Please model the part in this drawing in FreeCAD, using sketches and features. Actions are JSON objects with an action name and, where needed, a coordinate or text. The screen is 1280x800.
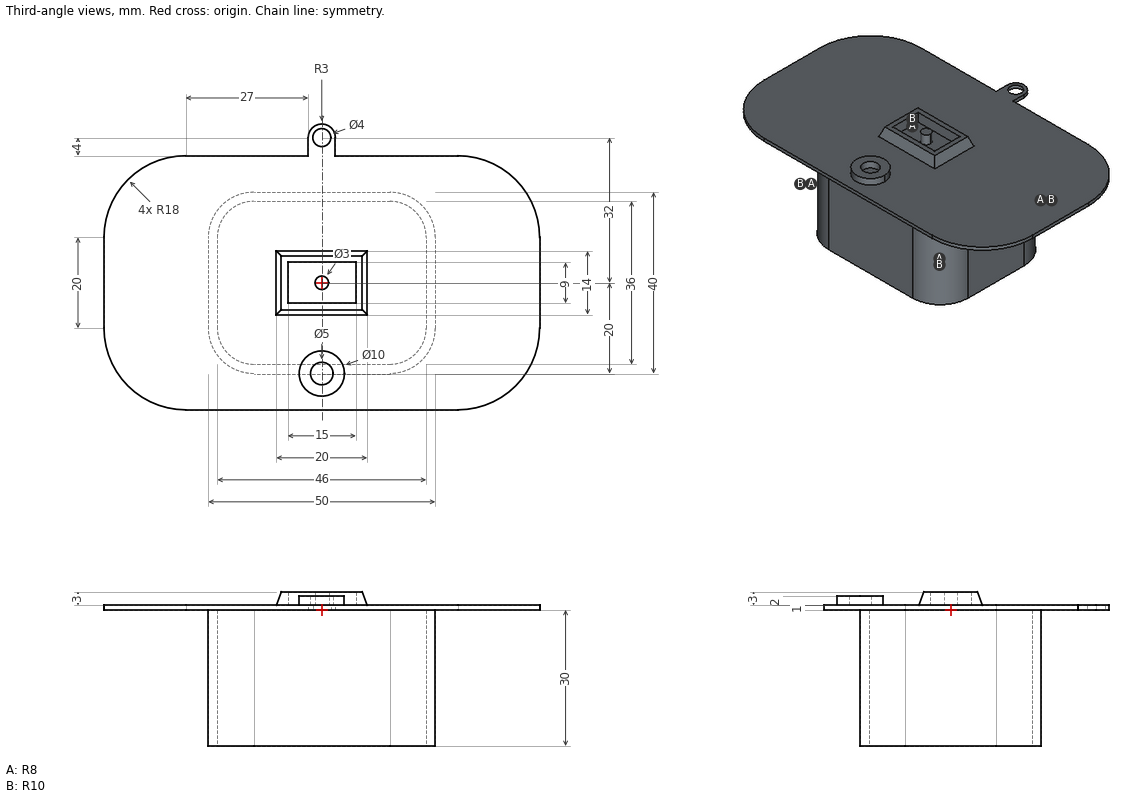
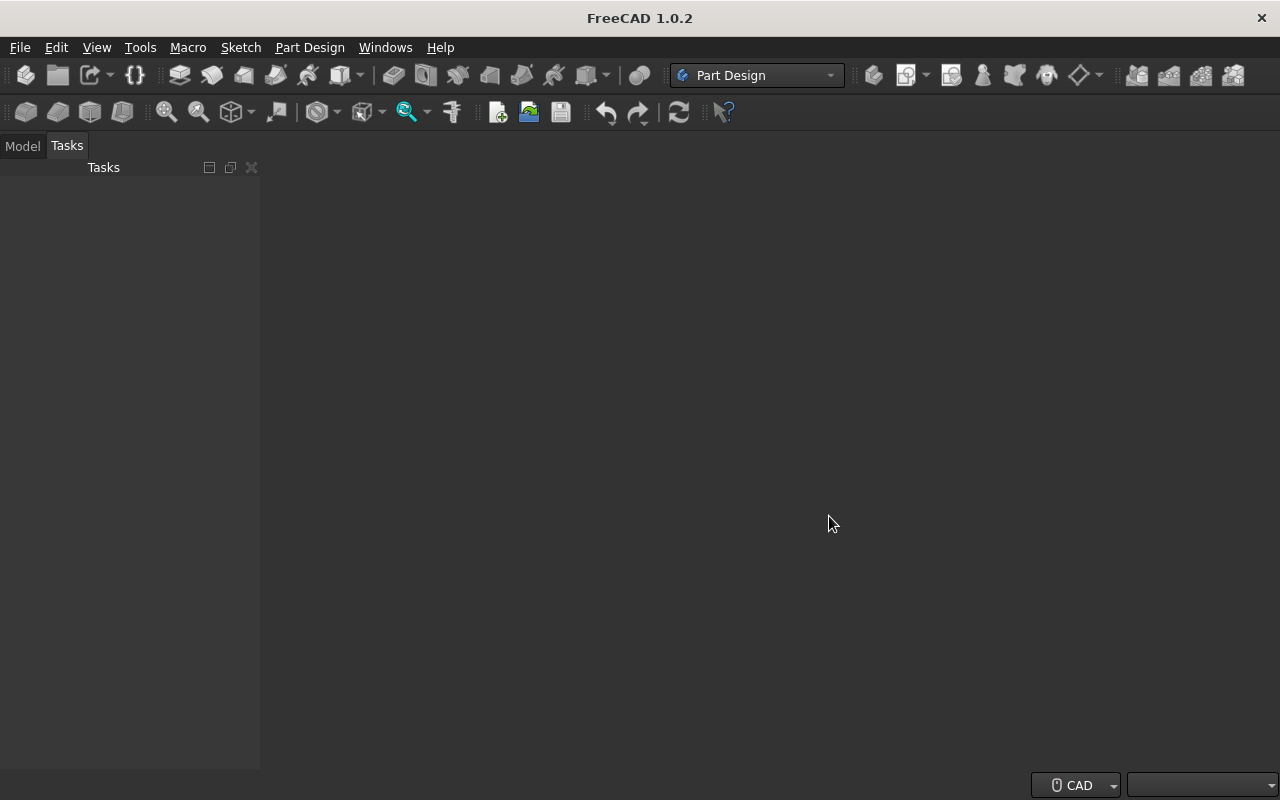
{"action": "left_click", "coordinate": [498, 112]}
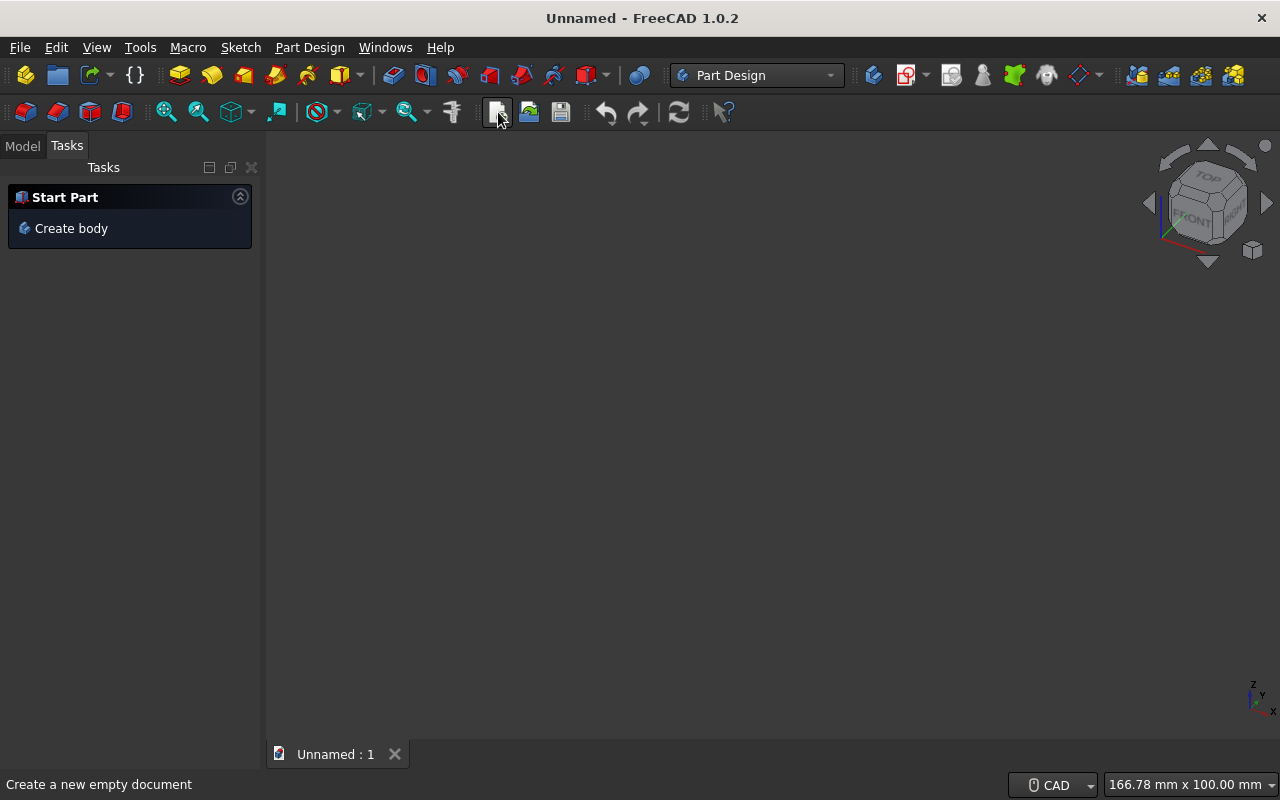
{"action": "left_click", "coordinate": [906, 76]}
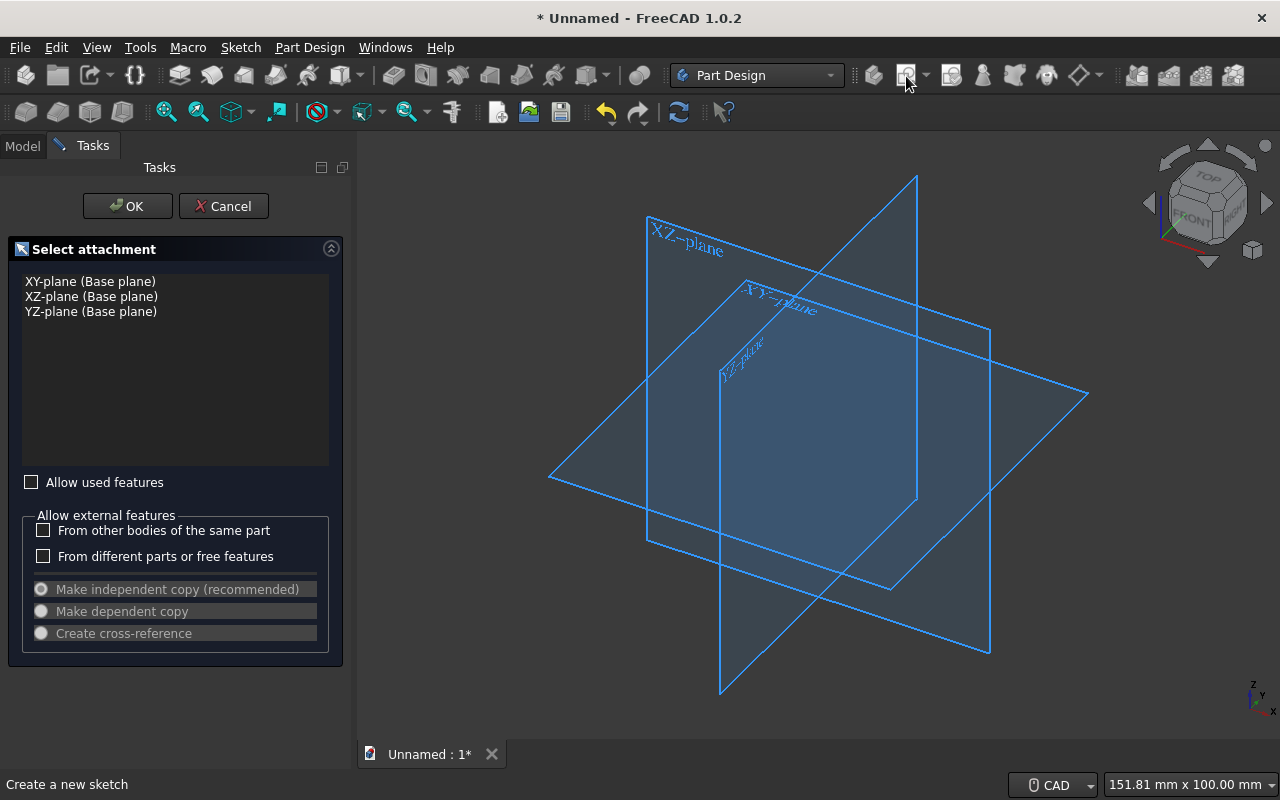
{"action": "left_click", "coordinate": [82, 282]}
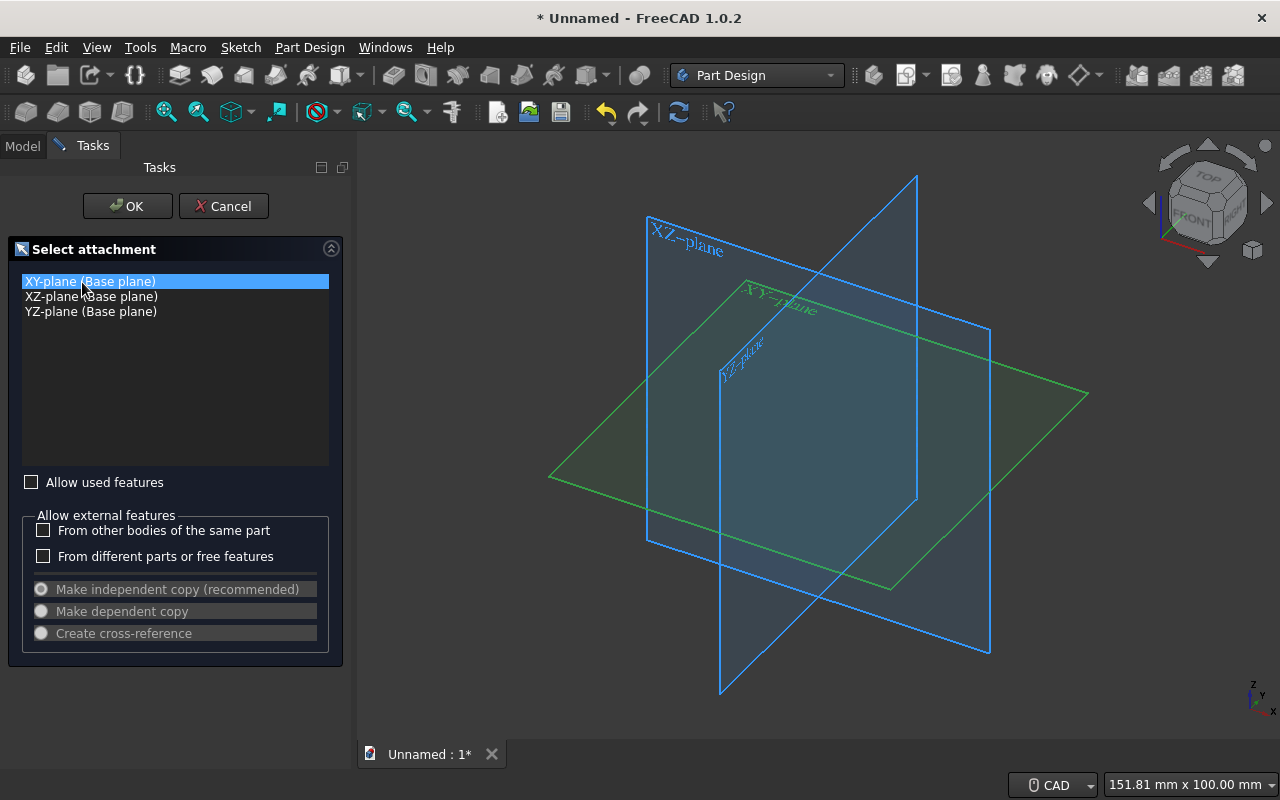
{"action": "left_click", "coordinate": [128, 206]}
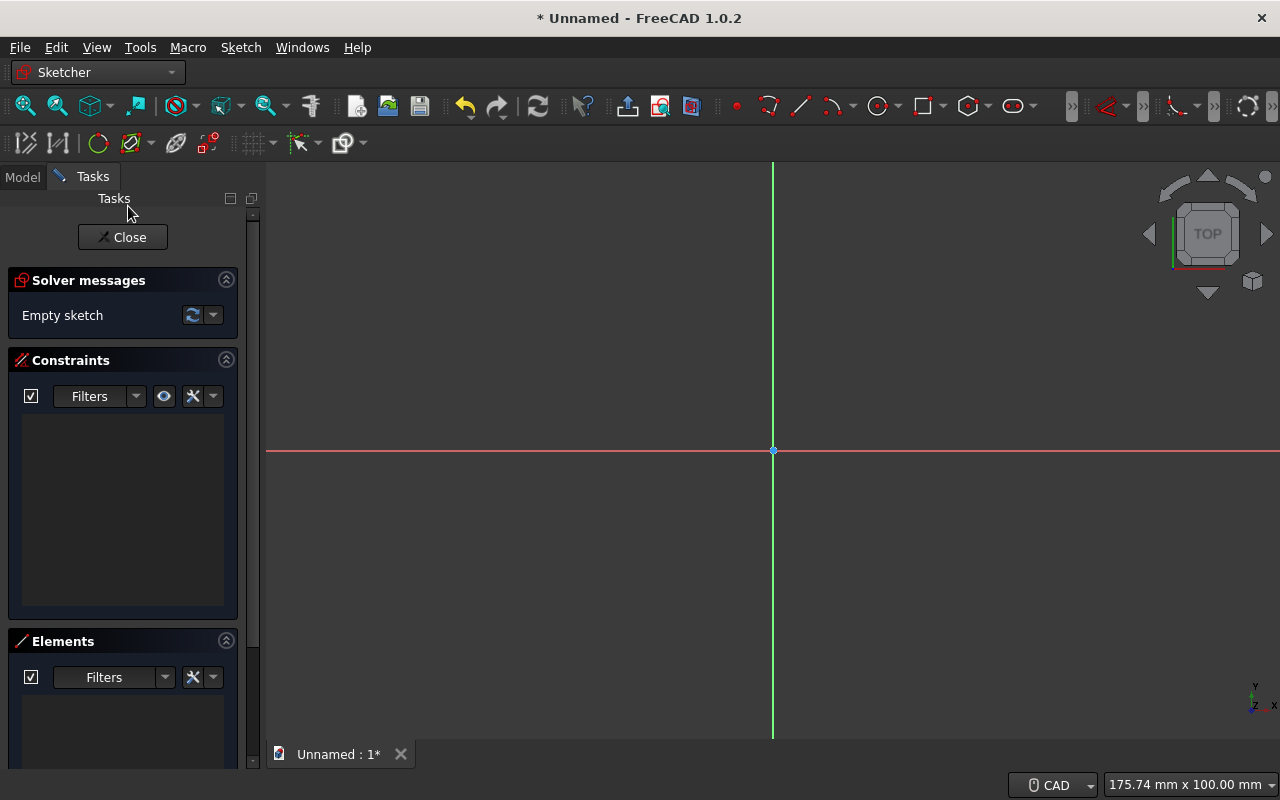
{"action": "left_click", "coordinate": [770, 106]}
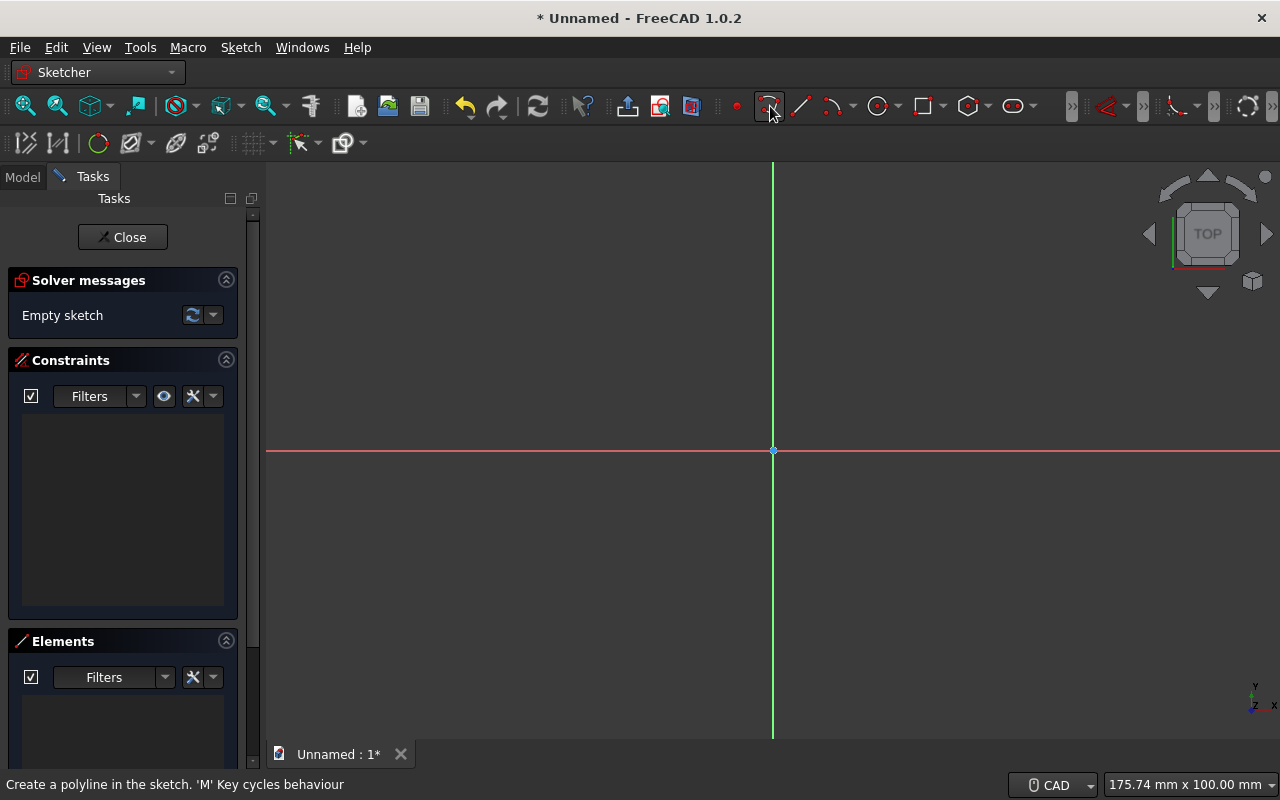
{"action": "left_click", "coordinate": [756, 266]}
{"action": "left_click", "coordinate": [756, 289]}
{"action": "left_click", "coordinate": [600, 289]}
{"action": "right_click", "coordinate": [600, 289]}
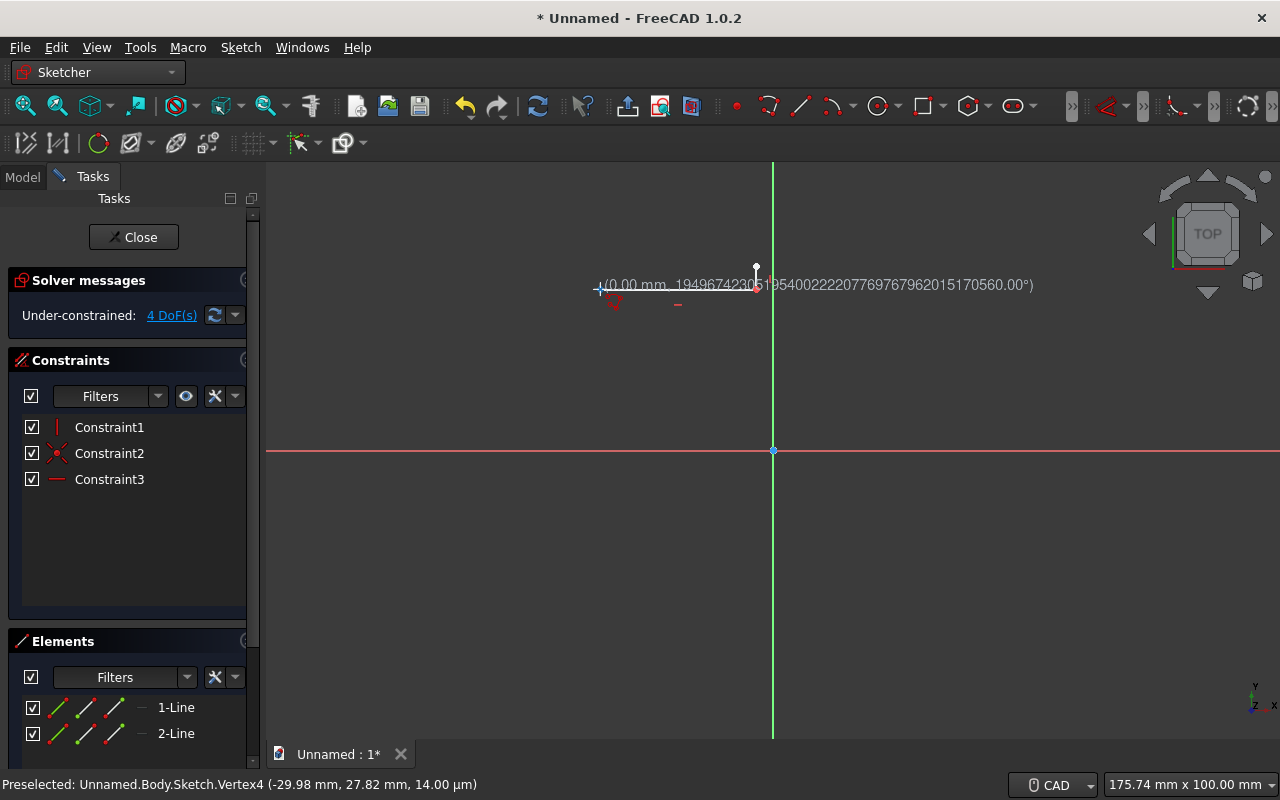
{"action": "left_click", "coordinate": [802, 106]}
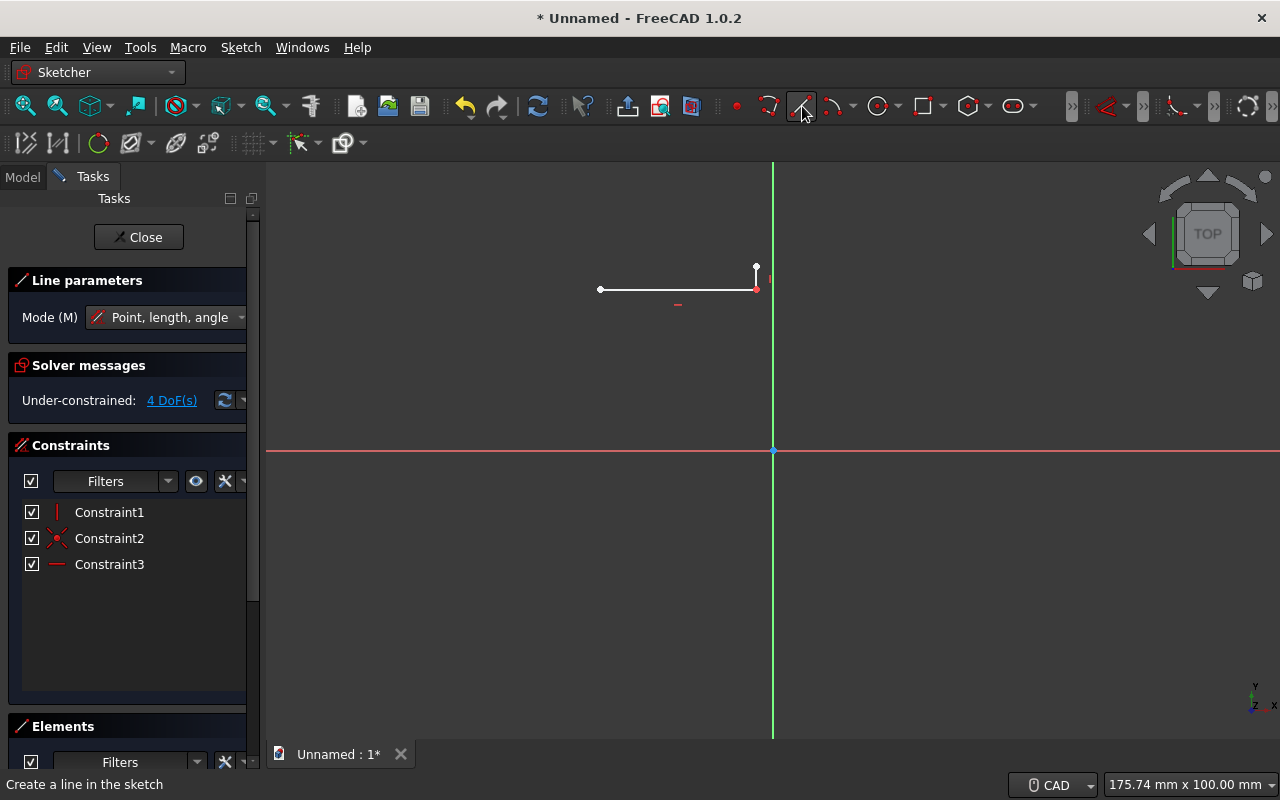
{"action": "left_click", "coordinate": [496, 393]}
{"action": "left_click", "coordinate": [496, 508]}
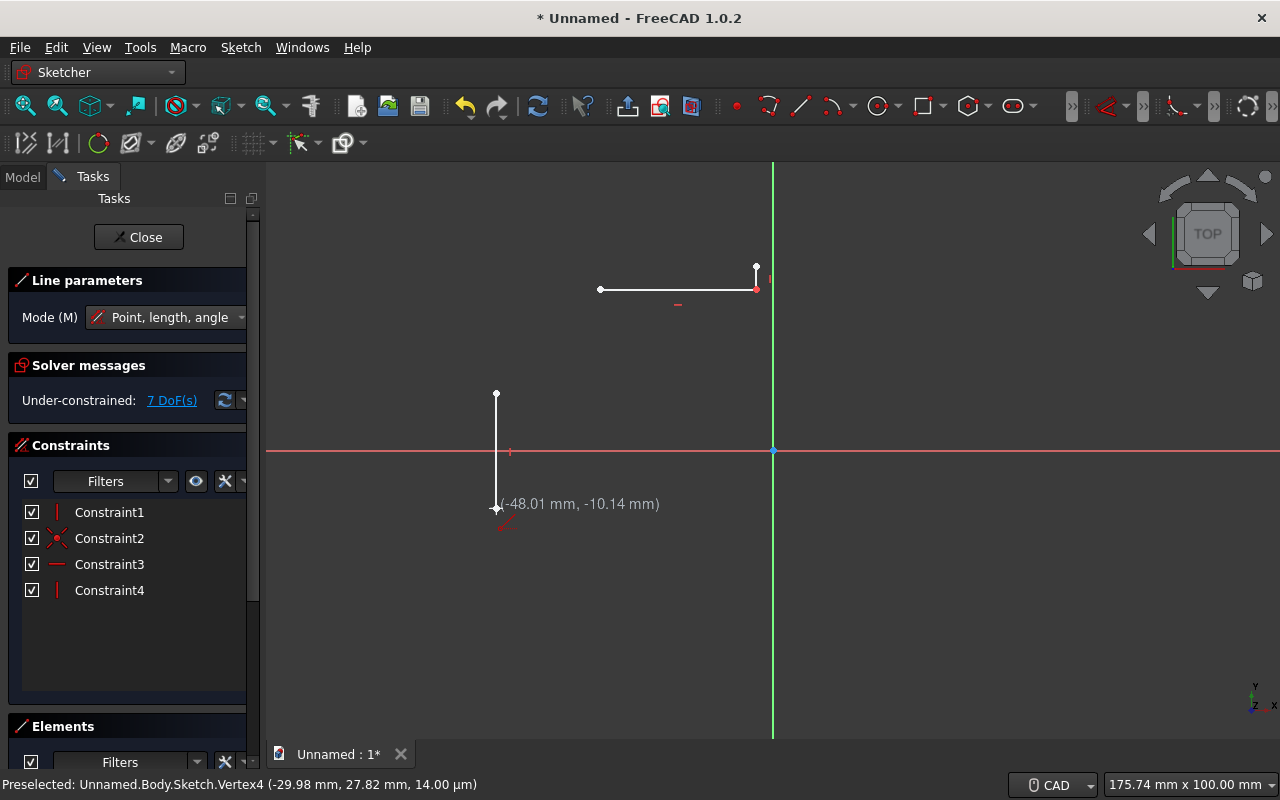
{"action": "left_click", "coordinate": [600, 612]}
{"action": "left_click", "coordinate": [946, 612]}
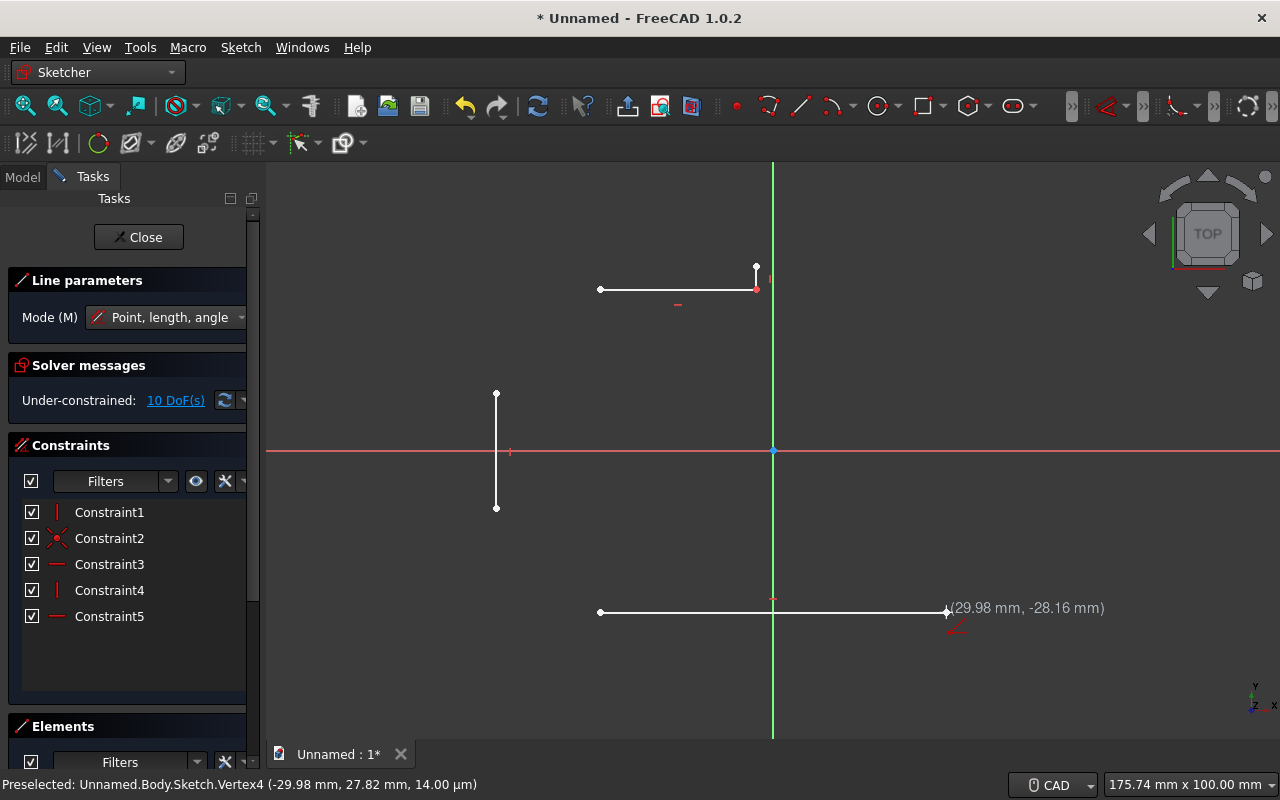
{"action": "left_click", "coordinate": [1050, 508]}
{"action": "left_click", "coordinate": [1050, 393]}